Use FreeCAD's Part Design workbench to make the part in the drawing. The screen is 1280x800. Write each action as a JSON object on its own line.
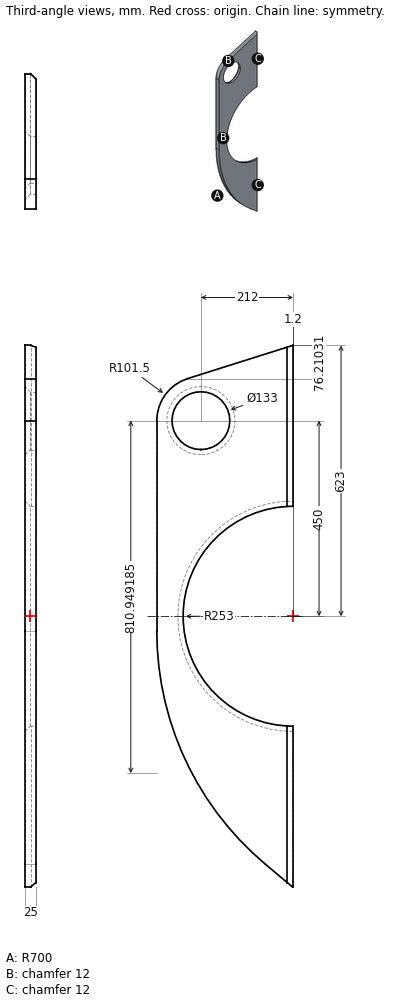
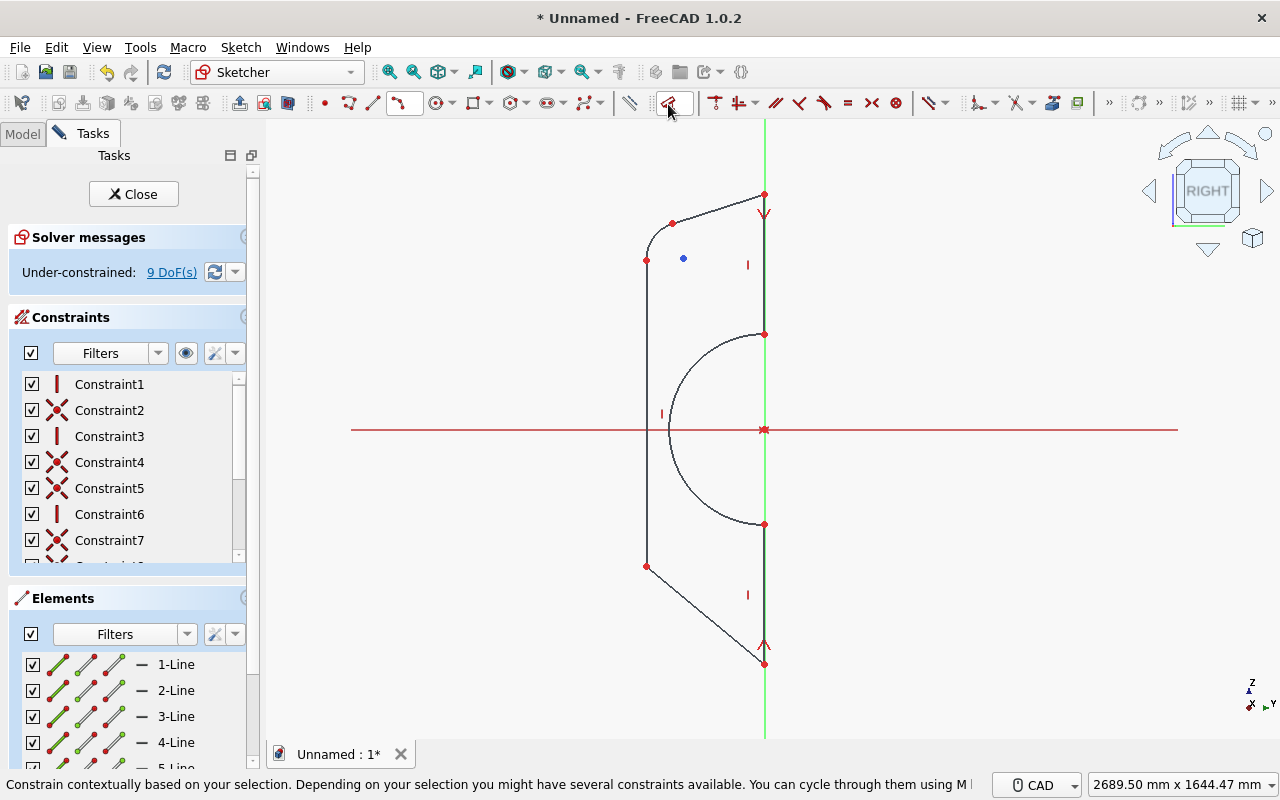
{"action": "left_click", "coordinate": [660, 231]}
{"action": "left_click", "coordinate": [640, 206]}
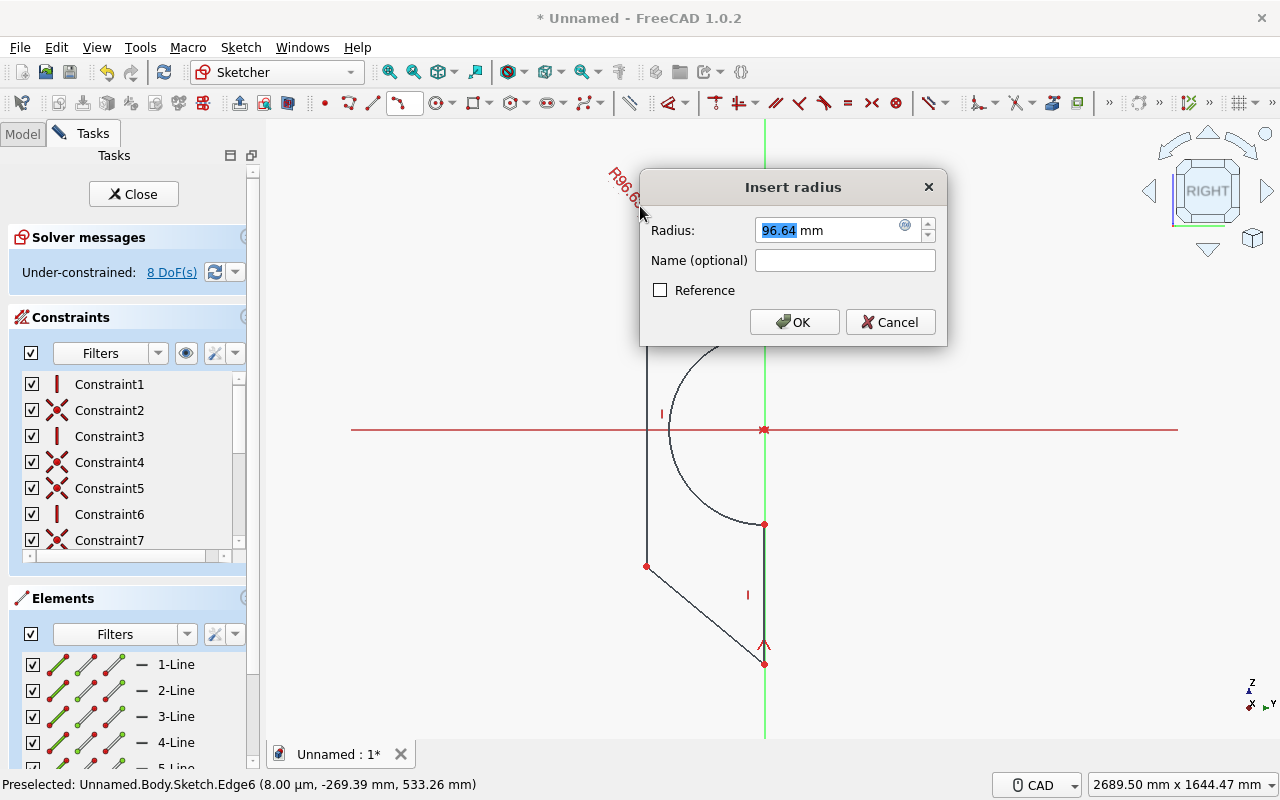
{"action": "type", "text": "101.5"}
{"action": "key", "text": "Return"}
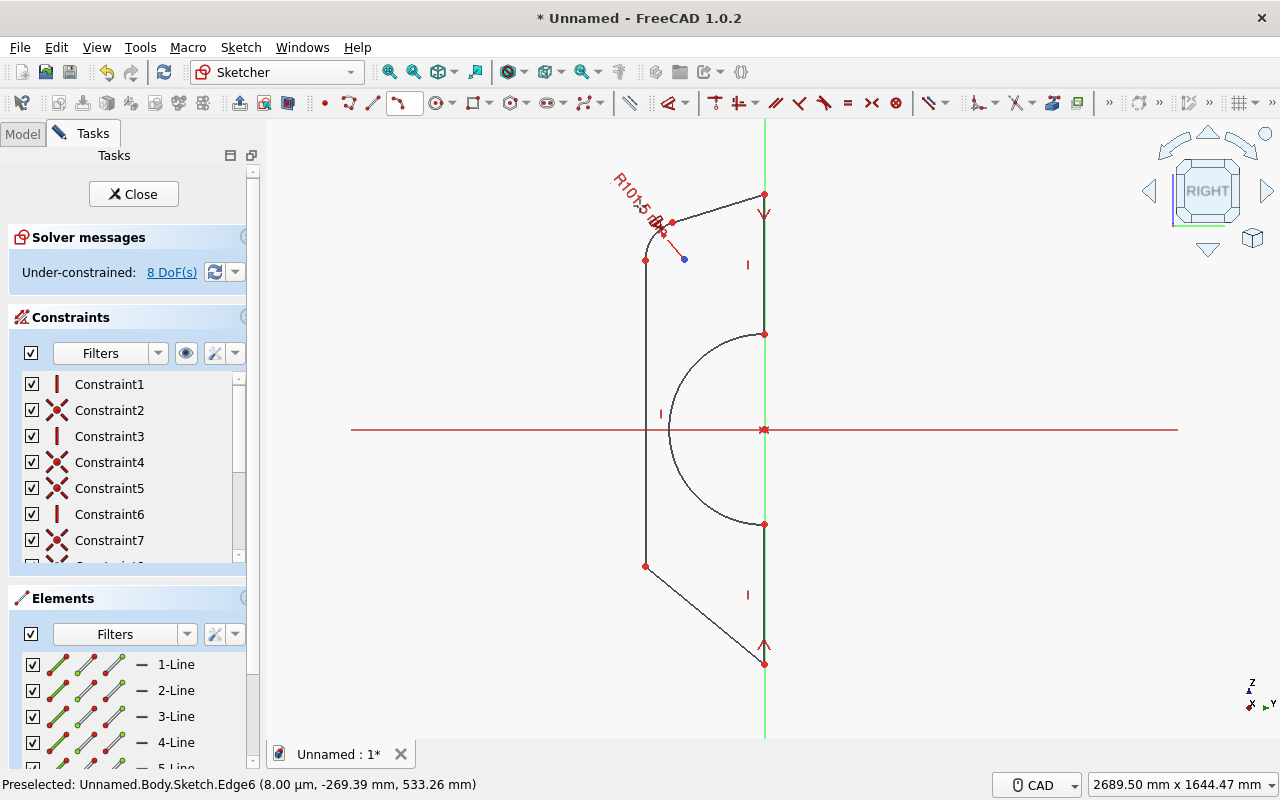
{"action": "left_click", "coordinate": [687, 374]}
{"action": "left_click", "coordinate": [661, 355]}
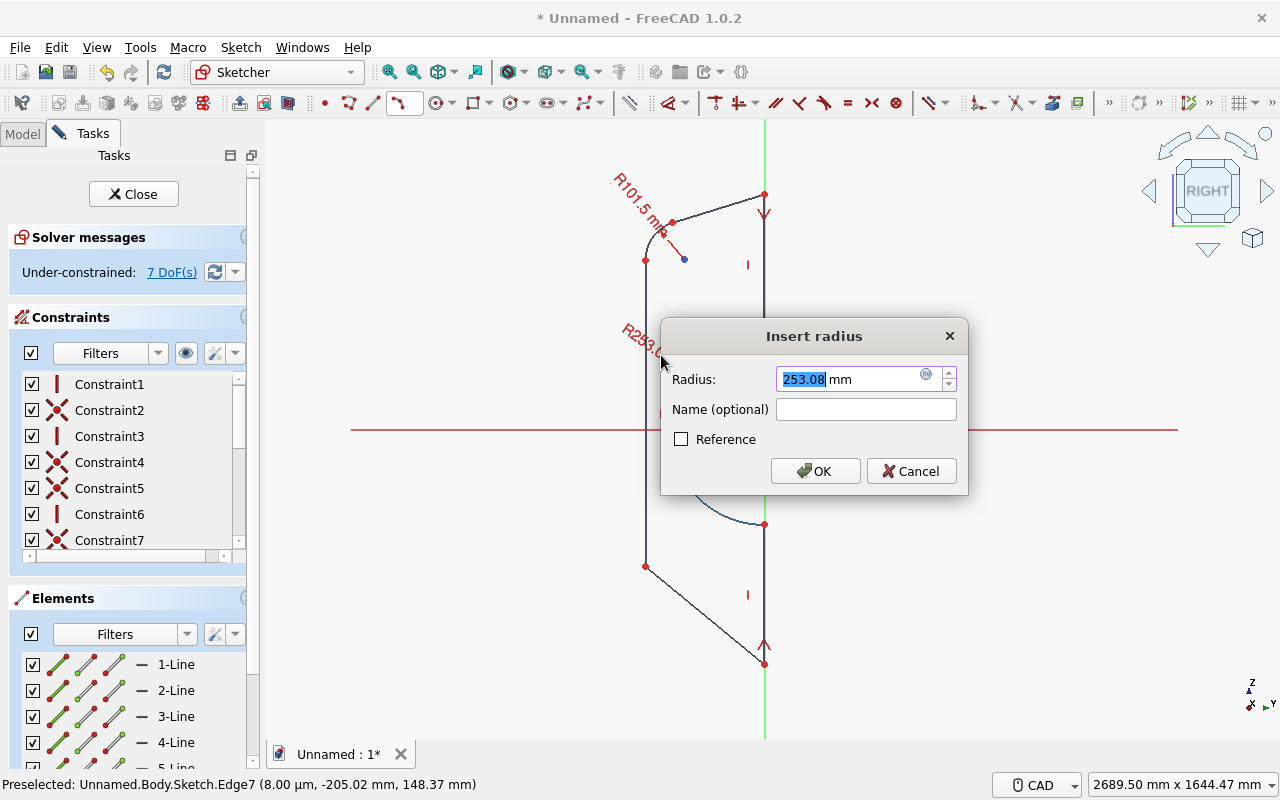
{"action": "type", "text": "253"}
{"action": "key", "text": "Return"}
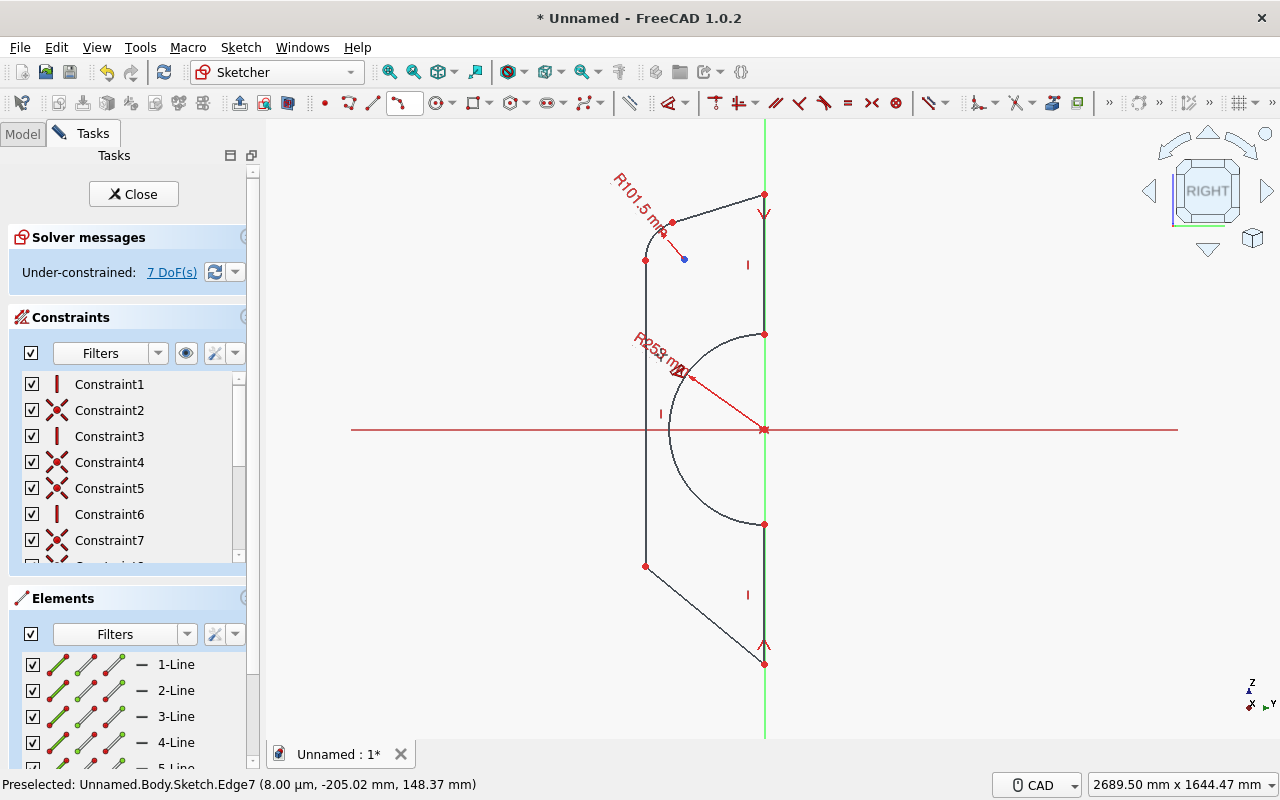
{"action": "scroll", "coordinate": [764, 334], "scroll_direction": "up", "scroll_amount": 23}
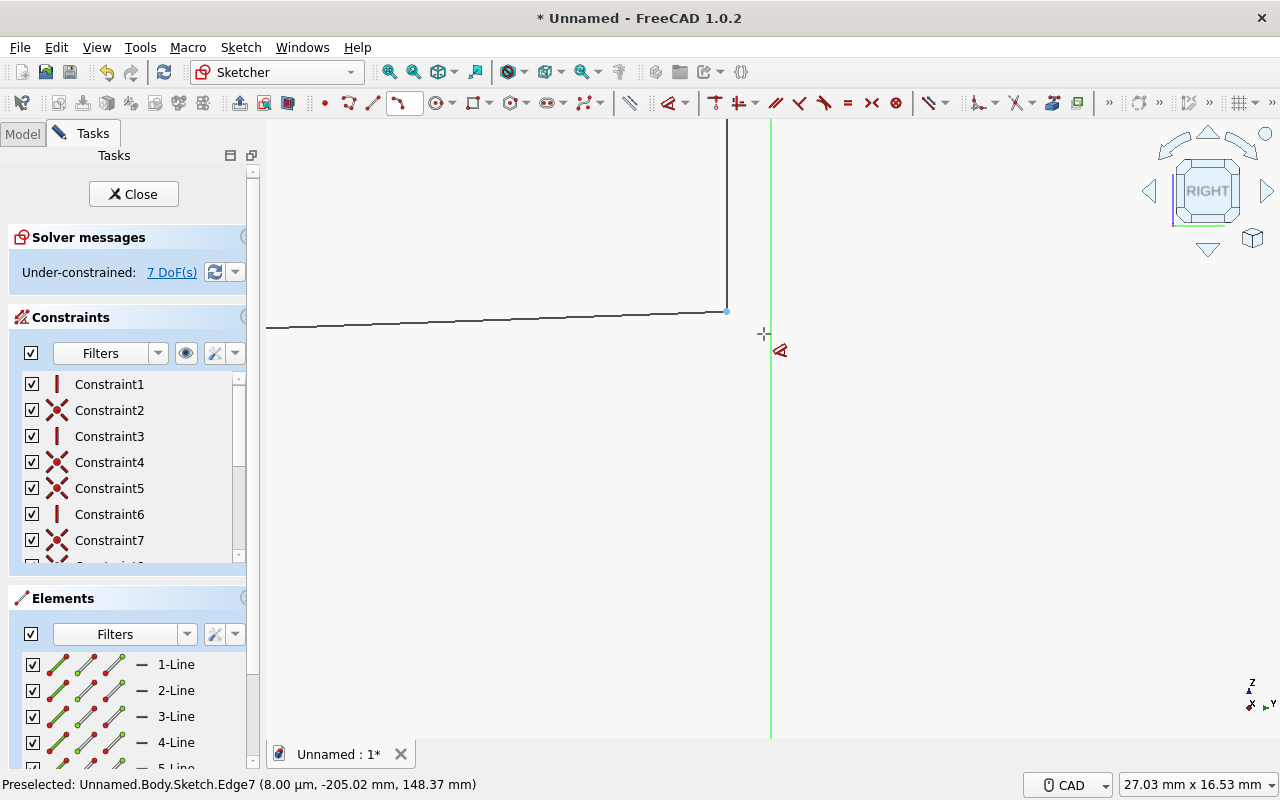
{"action": "left_click", "coordinate": [727, 312]}
{"action": "left_click", "coordinate": [749, 278]}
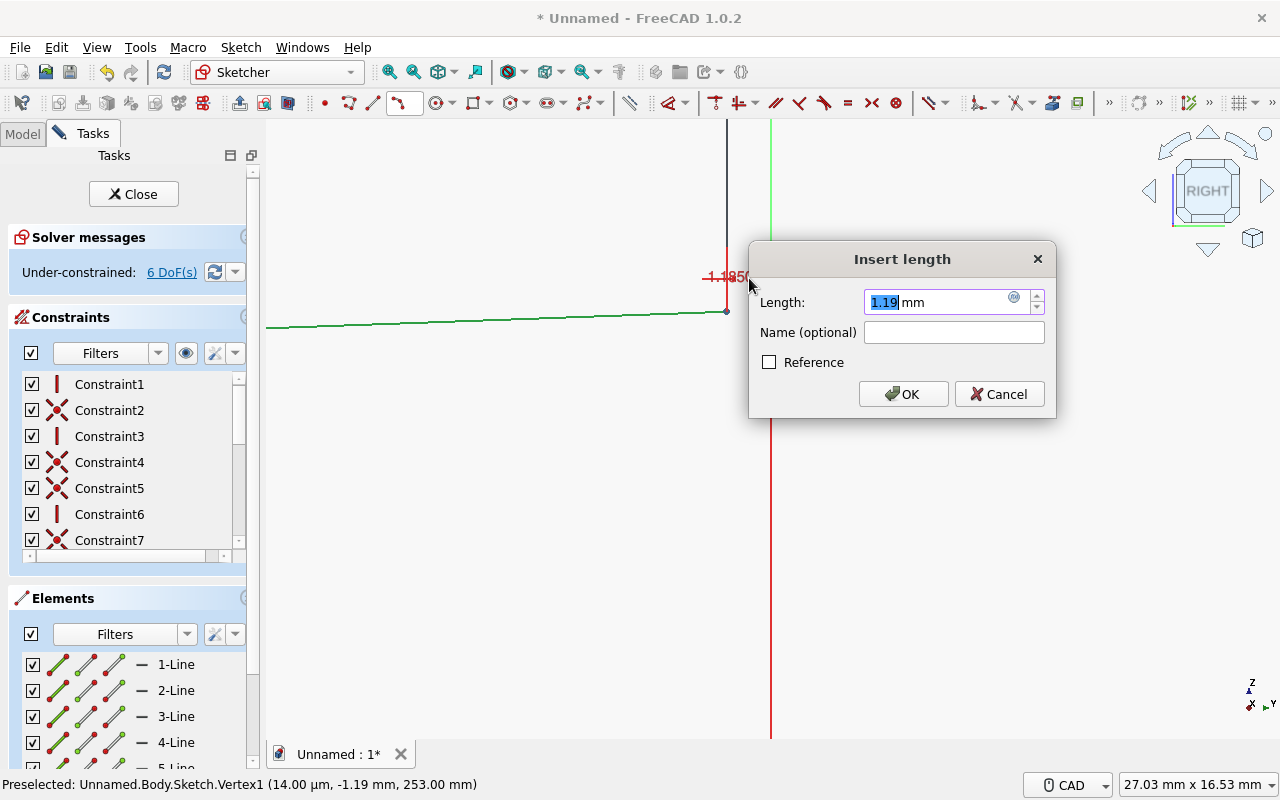
{"action": "type", "text": "1.2"}
{"action": "key", "text": "Return"}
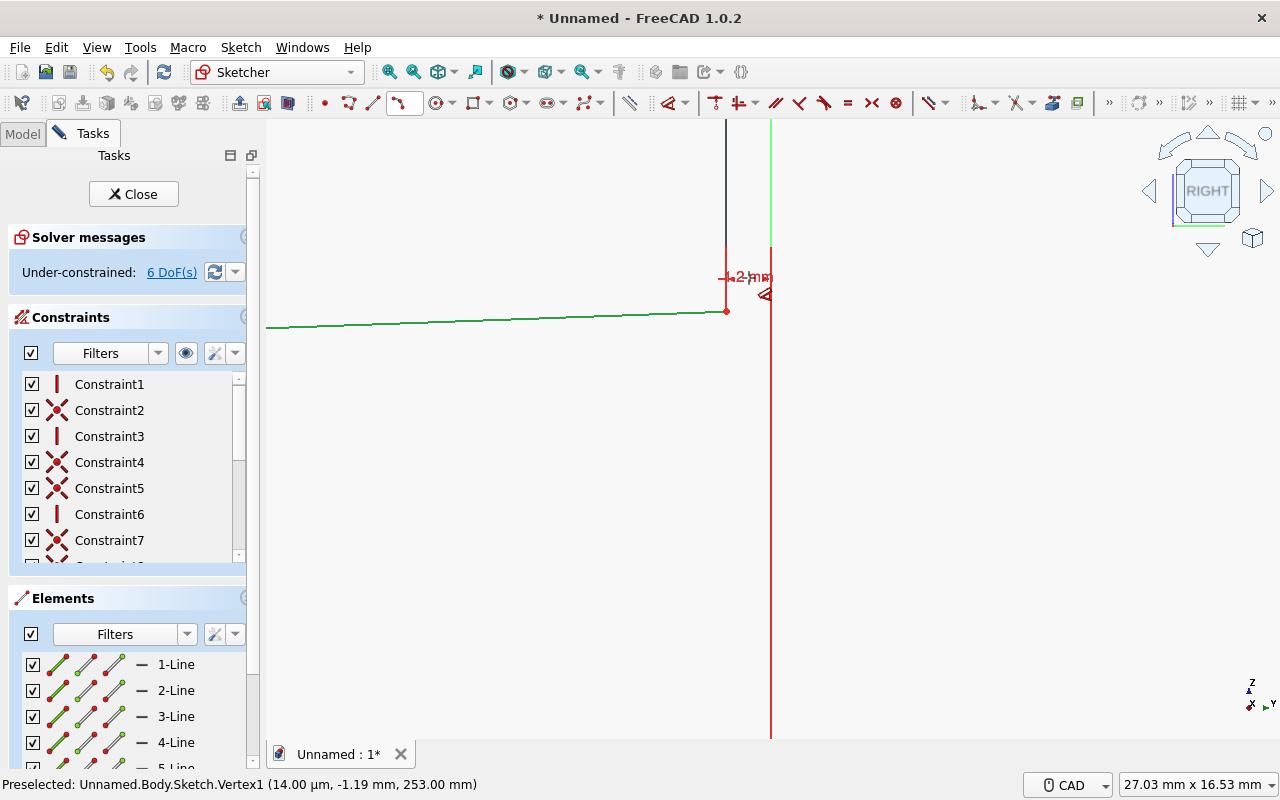
{"action": "scroll", "coordinate": [704, 429], "scroll_direction": "down", "scroll_amount": 15}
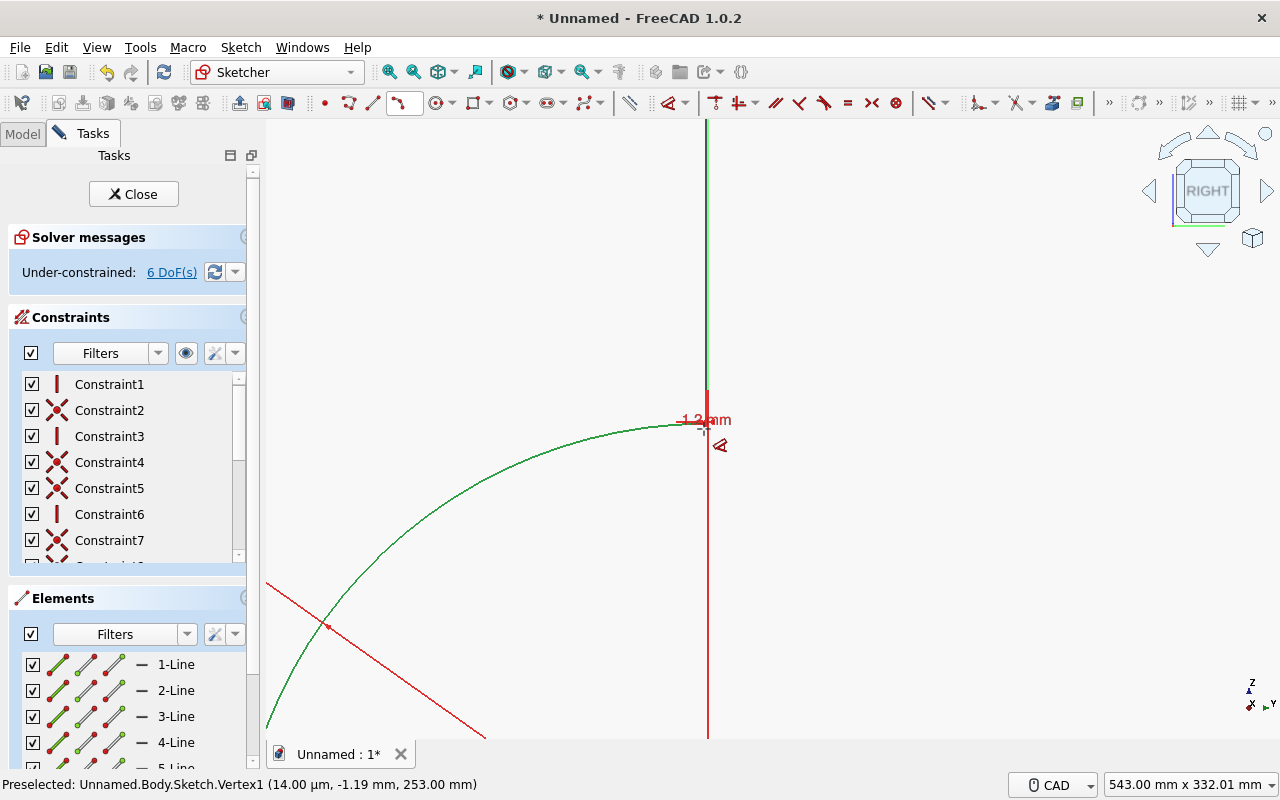
{"action": "scroll", "coordinate": [762, 337], "scroll_direction": "down", "scroll_amount": 9}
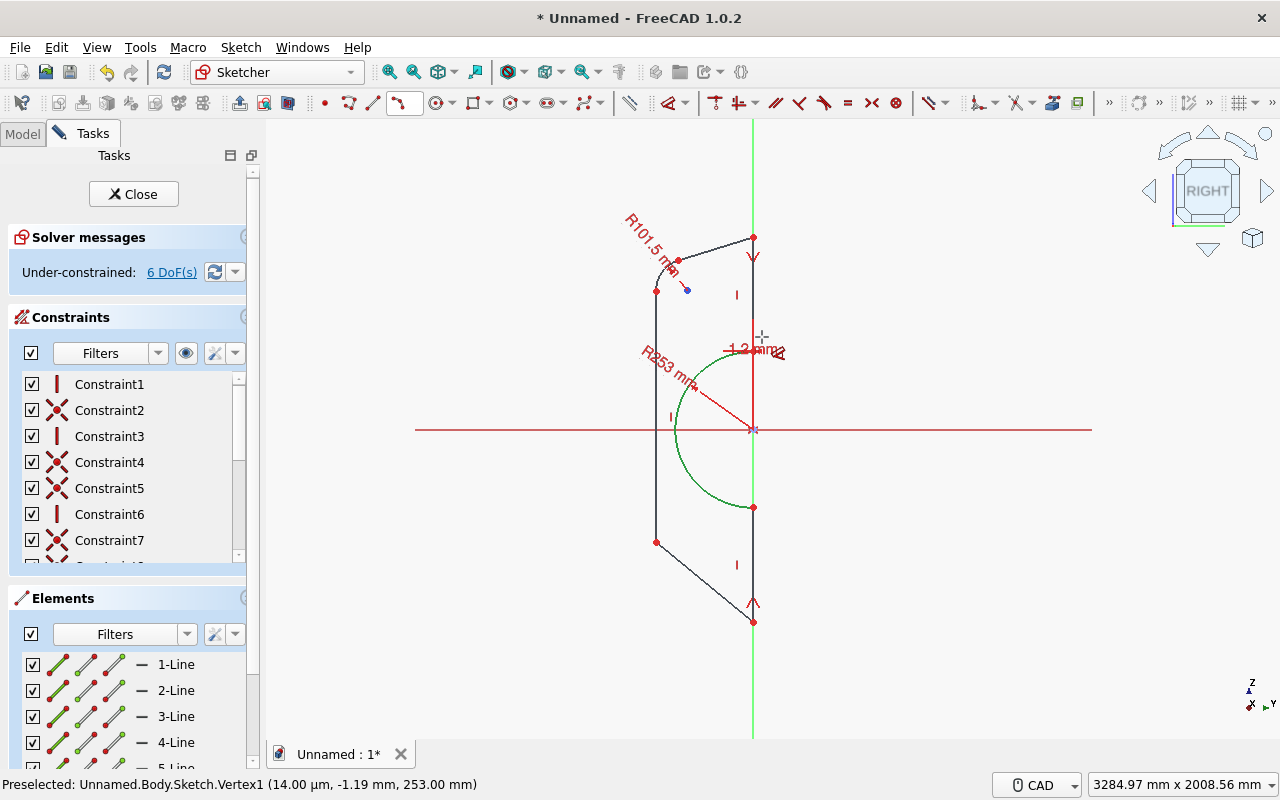
{"action": "left_click", "coordinate": [753, 237]}
{"action": "left_click", "coordinate": [787, 289]}